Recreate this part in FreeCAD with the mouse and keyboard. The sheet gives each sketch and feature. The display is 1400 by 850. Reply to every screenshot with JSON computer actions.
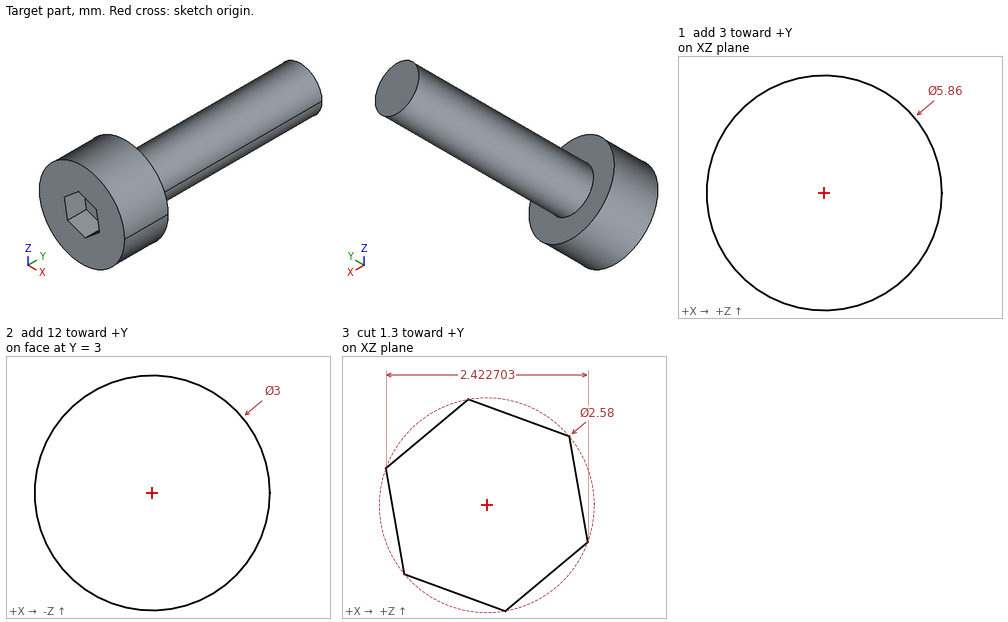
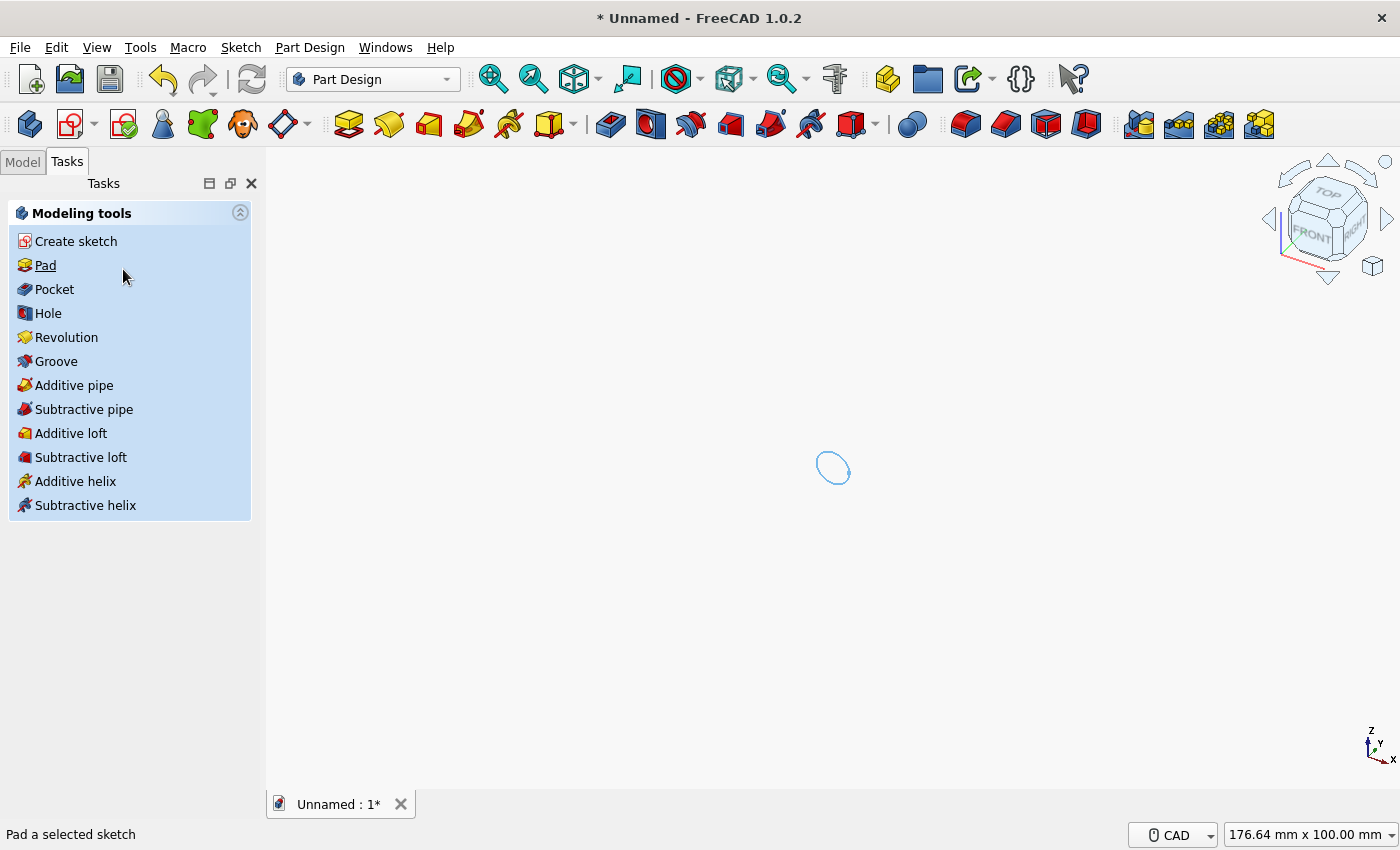
{"action": "left_click", "coordinate": [350, 124]}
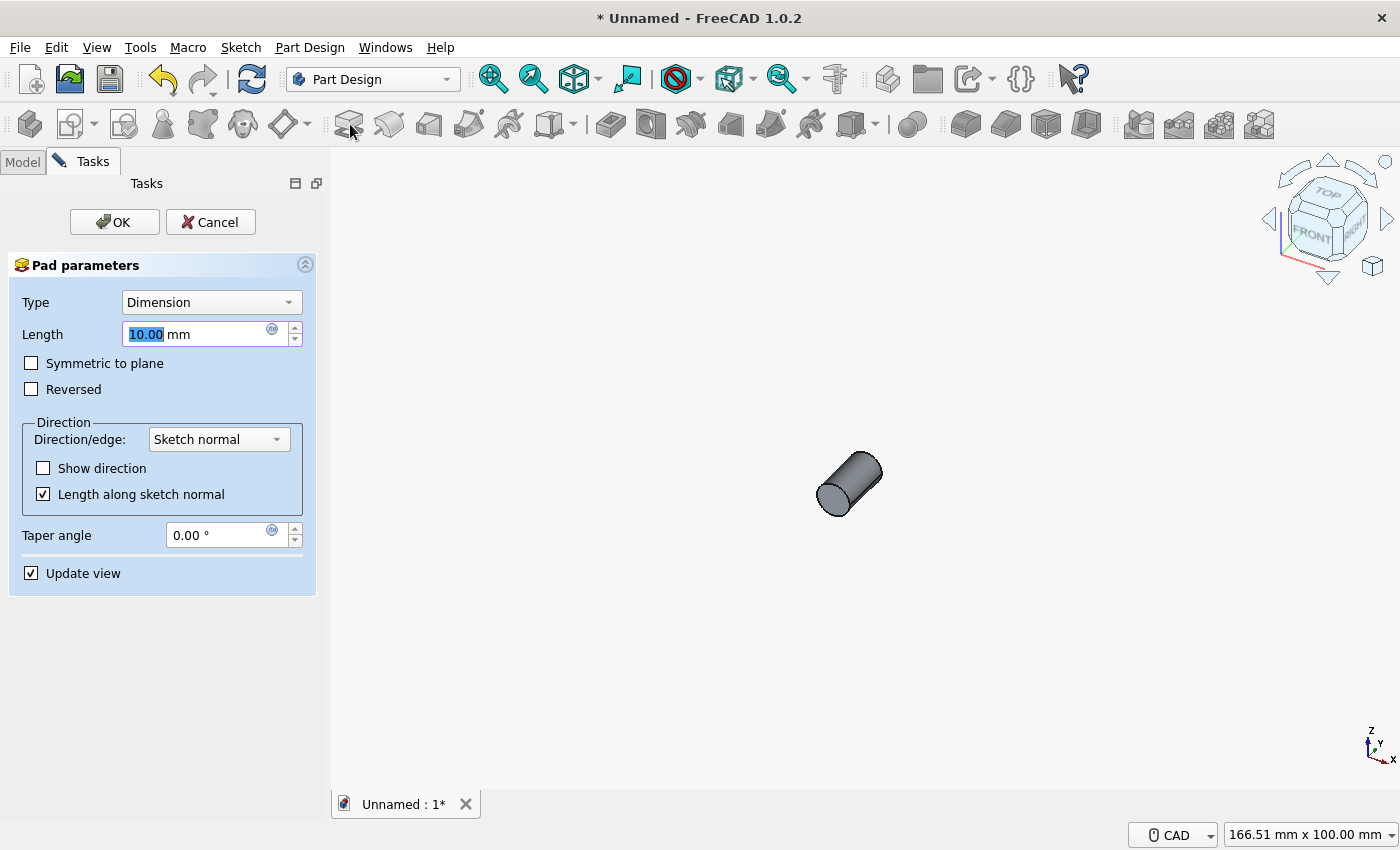
{"action": "type", "text": "3"}
{"action": "key", "text": "Tab"}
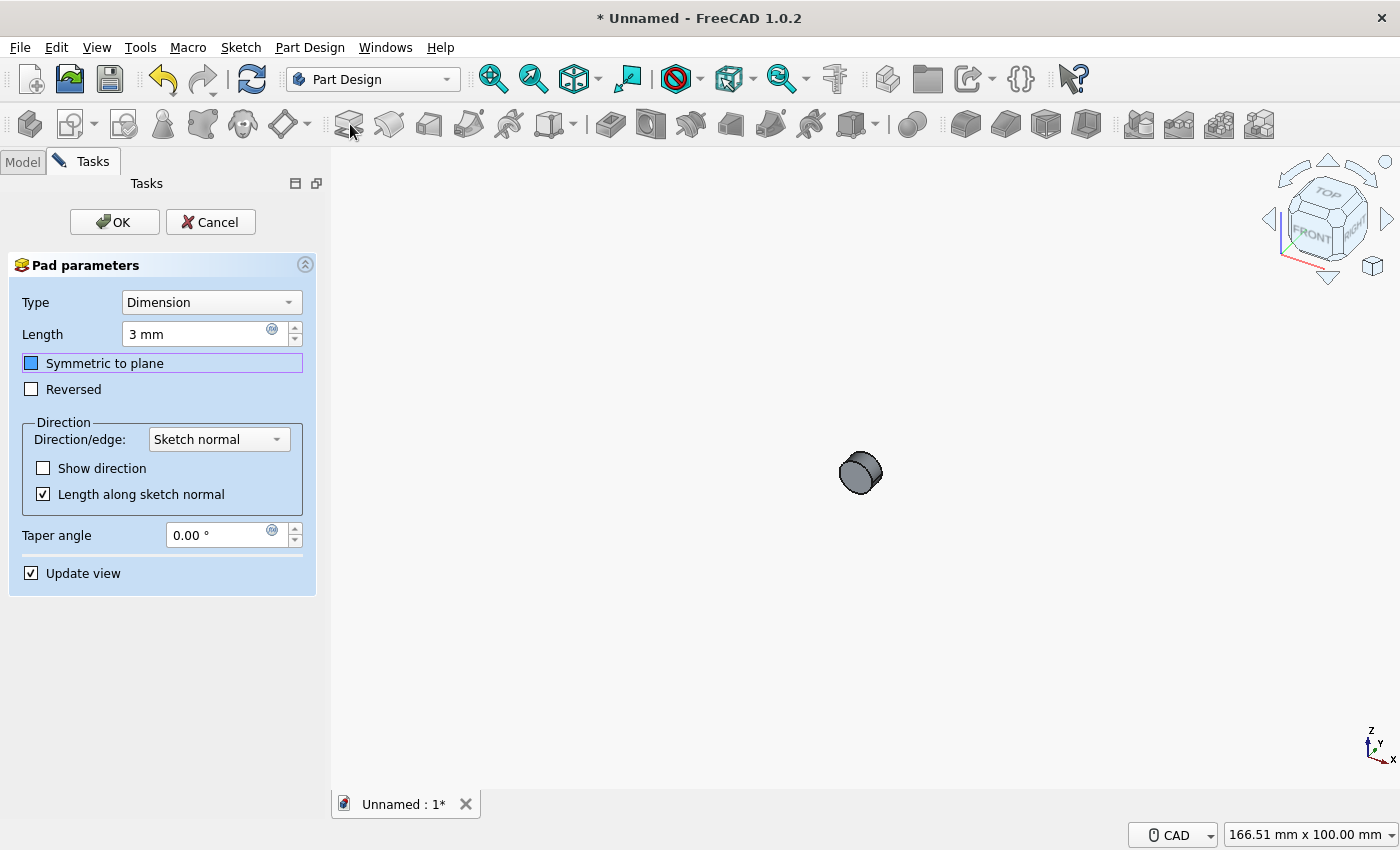
{"action": "left_click", "coordinate": [30, 389]}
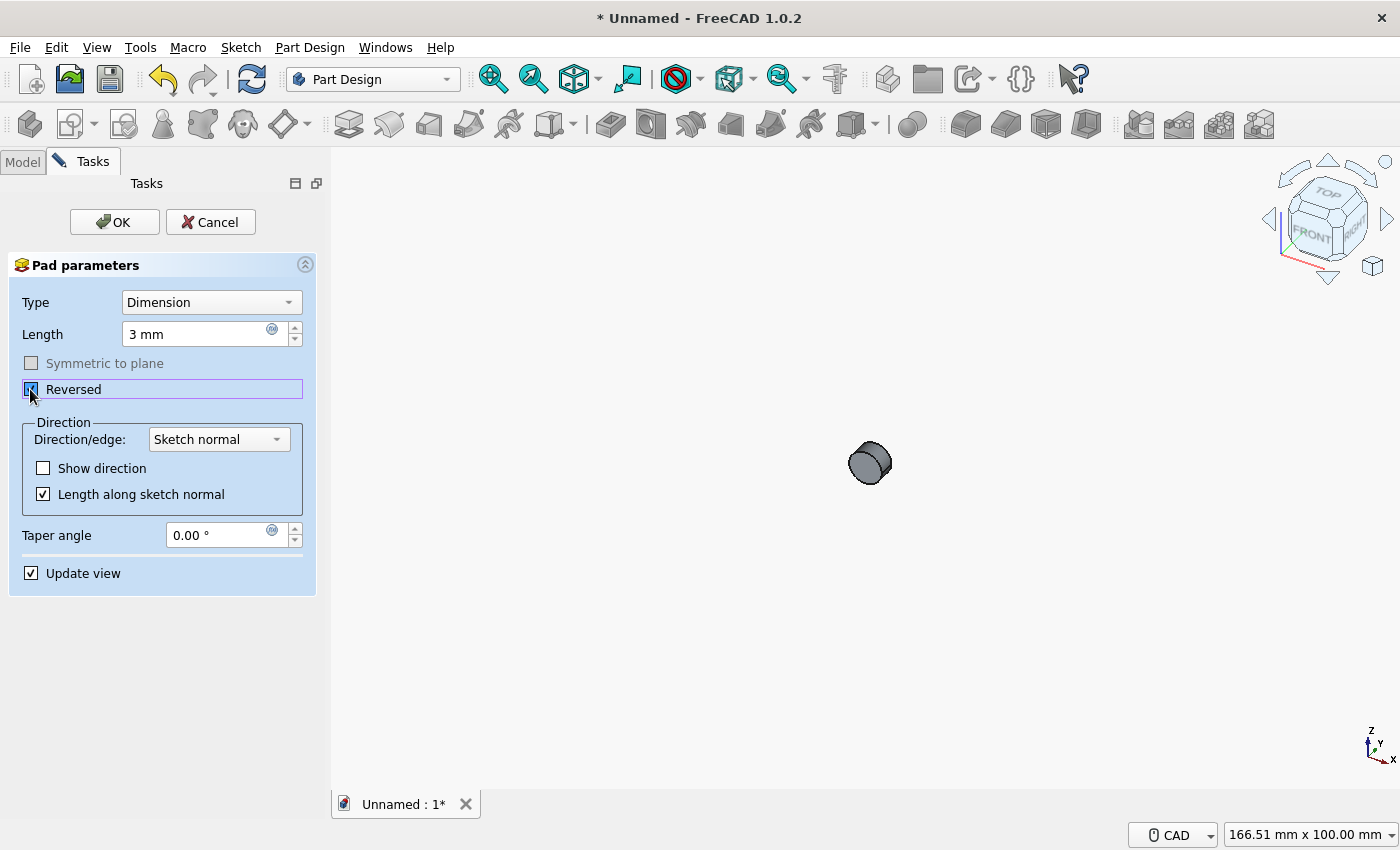
{"action": "left_click", "coordinate": [115, 222]}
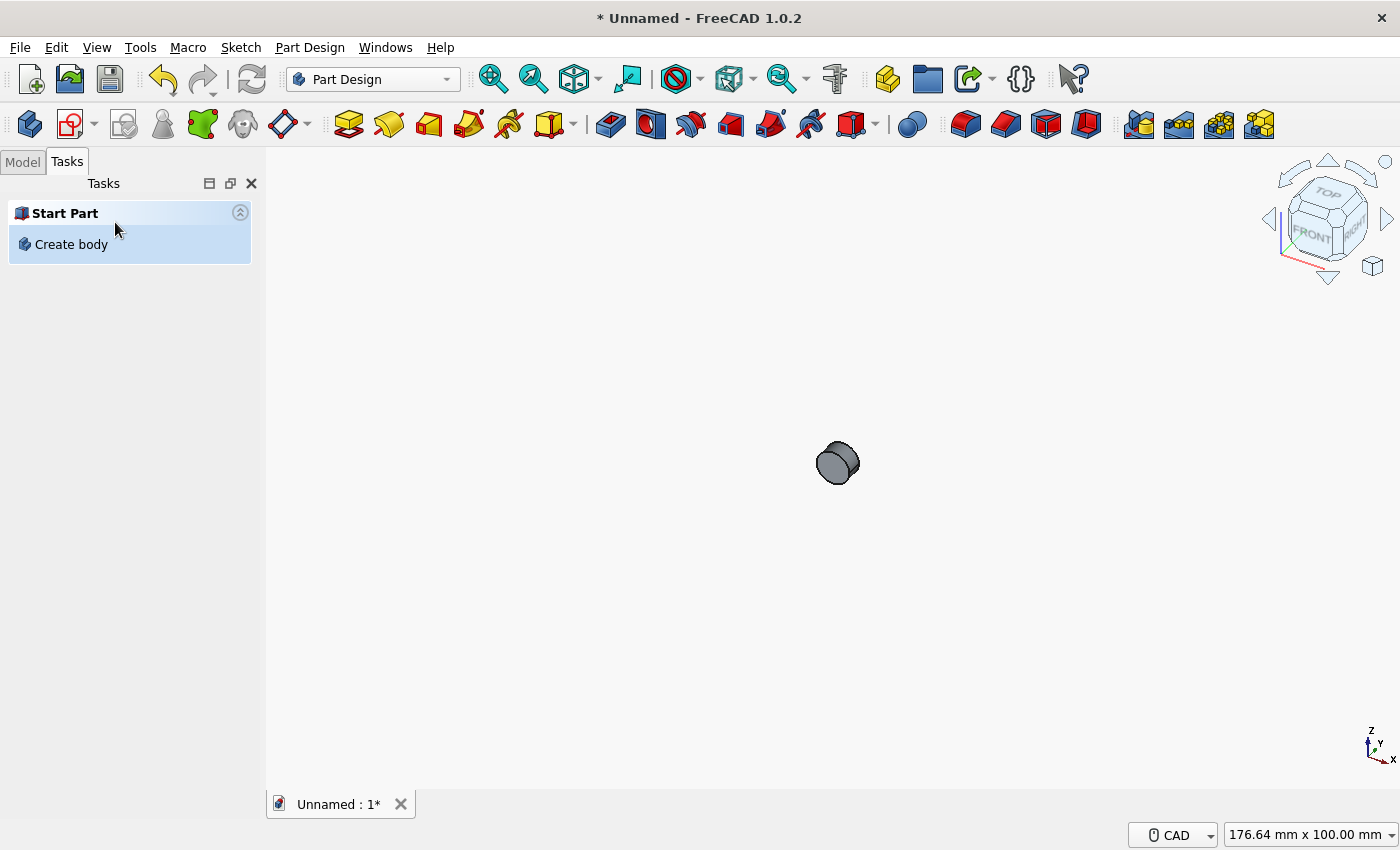
{"action": "left_click", "coordinate": [494, 80]}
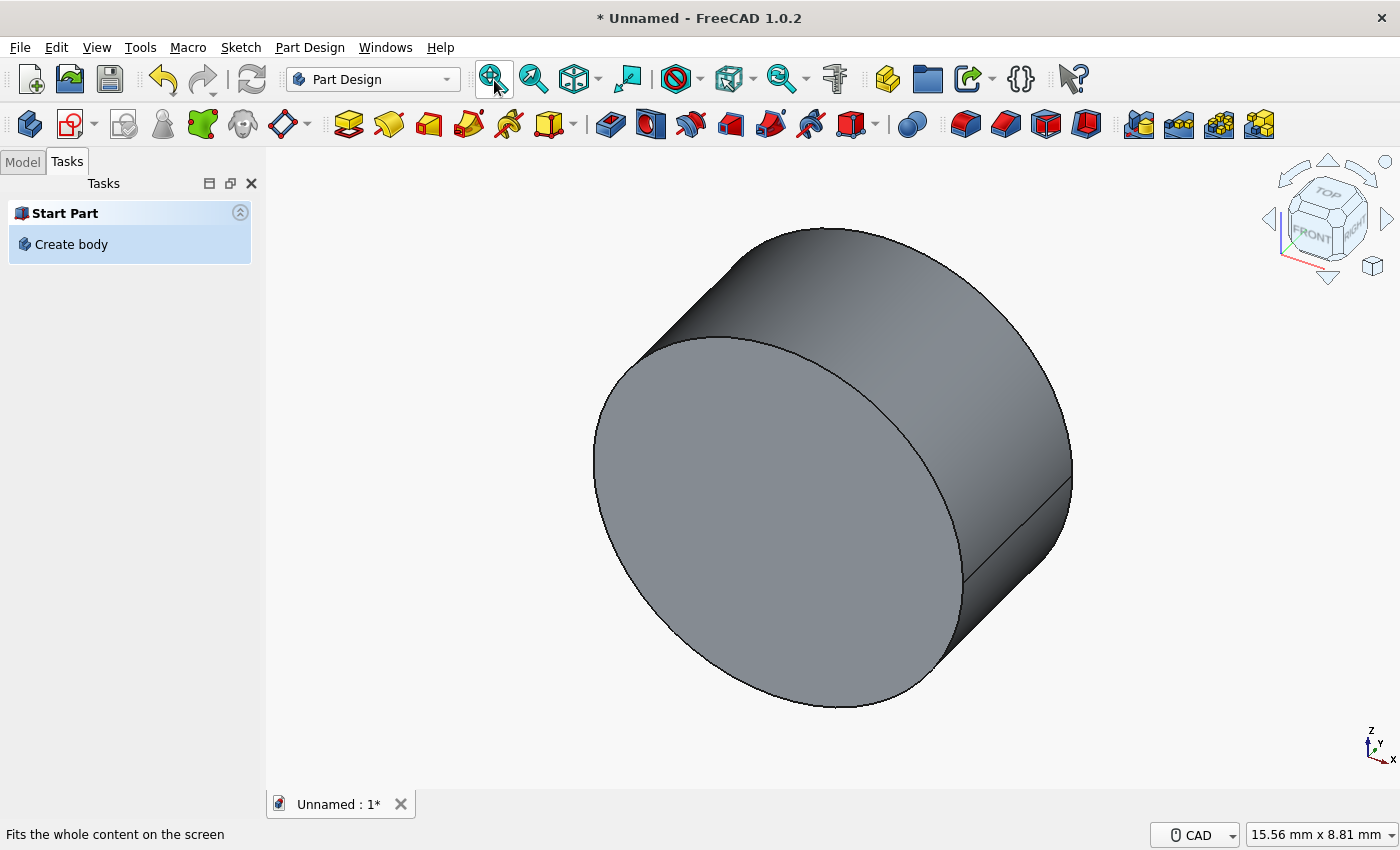
{"action": "key", "text": "4"}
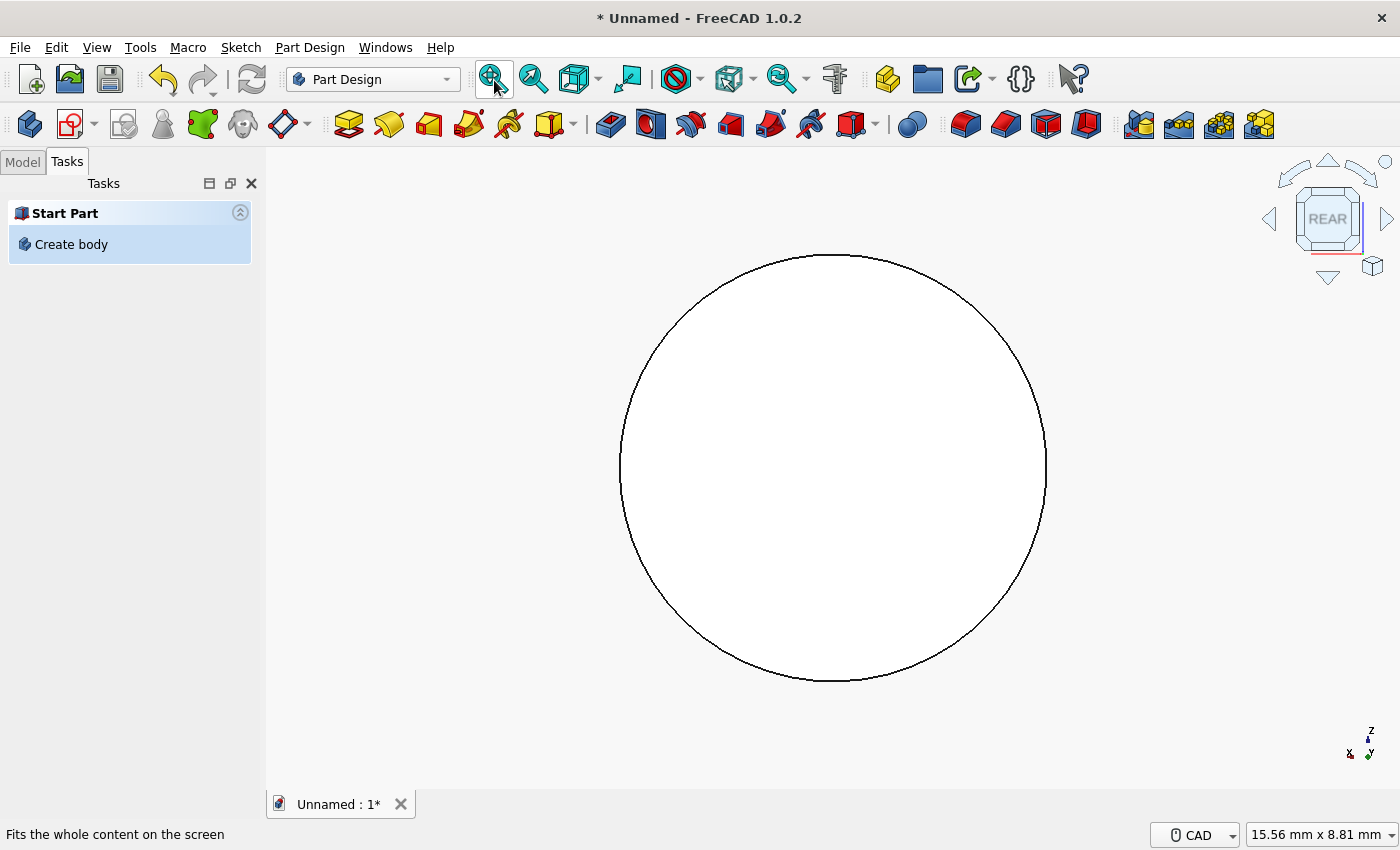
{"action": "left_click", "coordinate": [833, 467]}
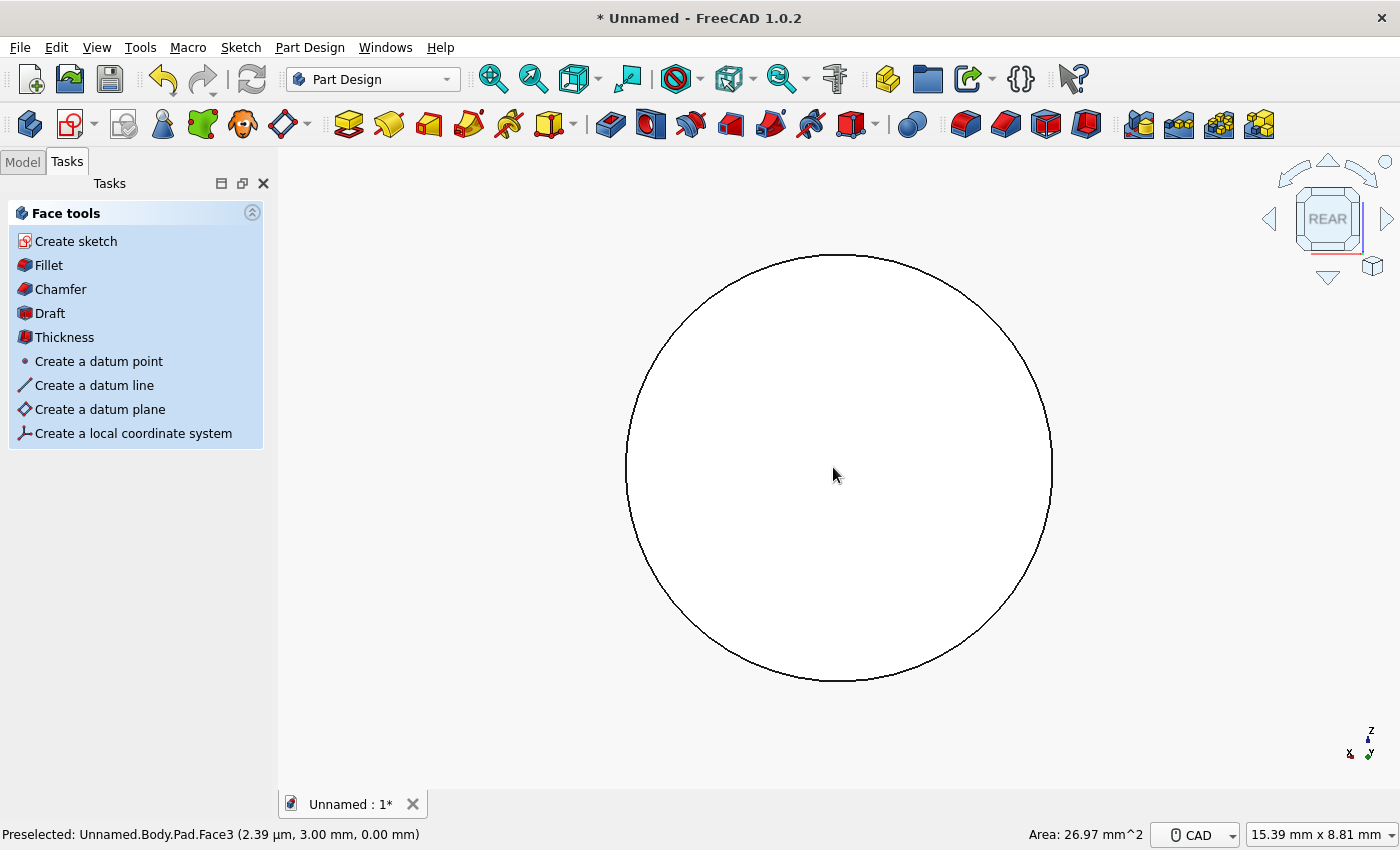
{"action": "left_click", "coordinate": [70, 124]}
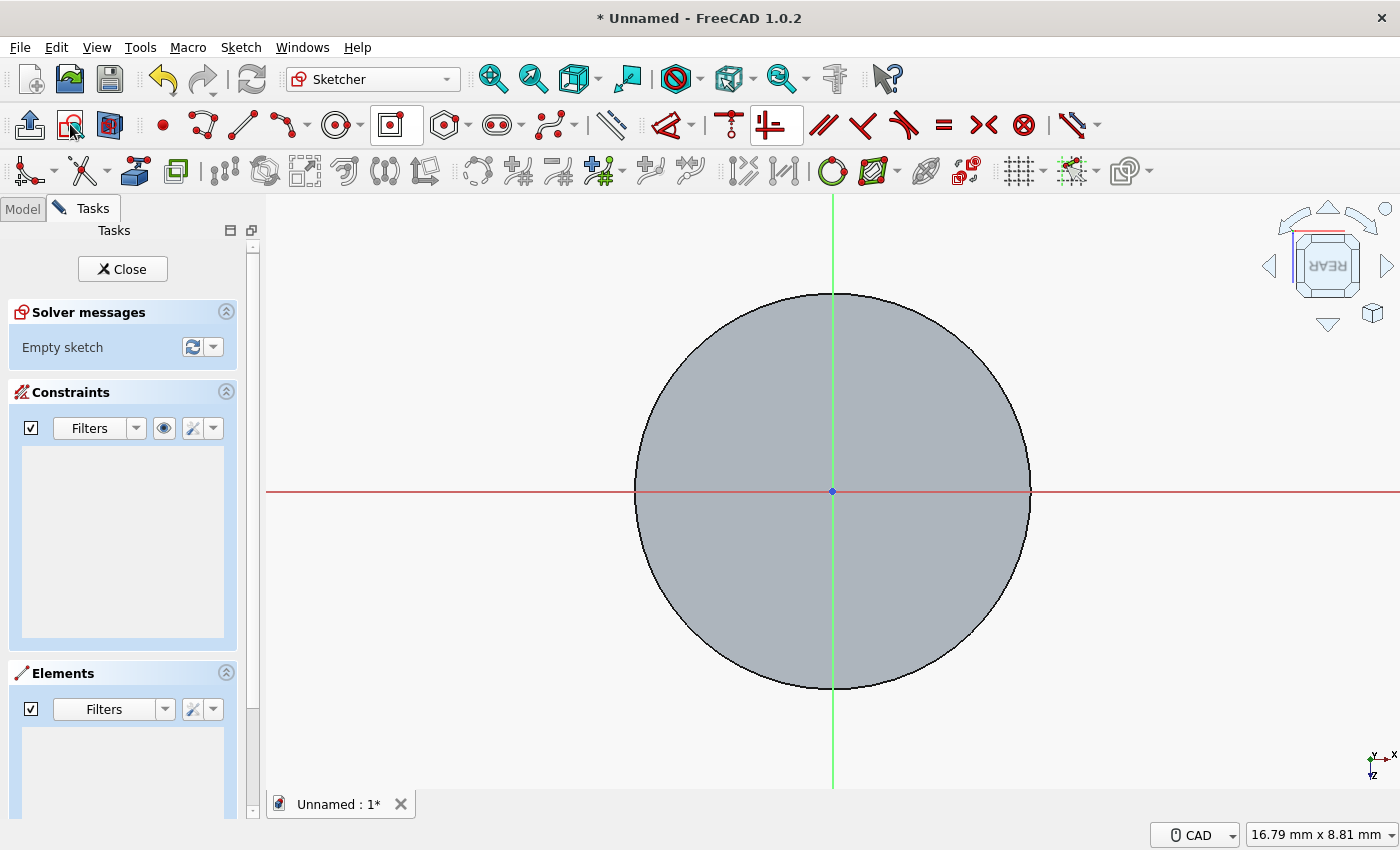
{"action": "scroll", "coordinate": [916, 492], "scroll_direction": "up", "scroll_amount": 3}